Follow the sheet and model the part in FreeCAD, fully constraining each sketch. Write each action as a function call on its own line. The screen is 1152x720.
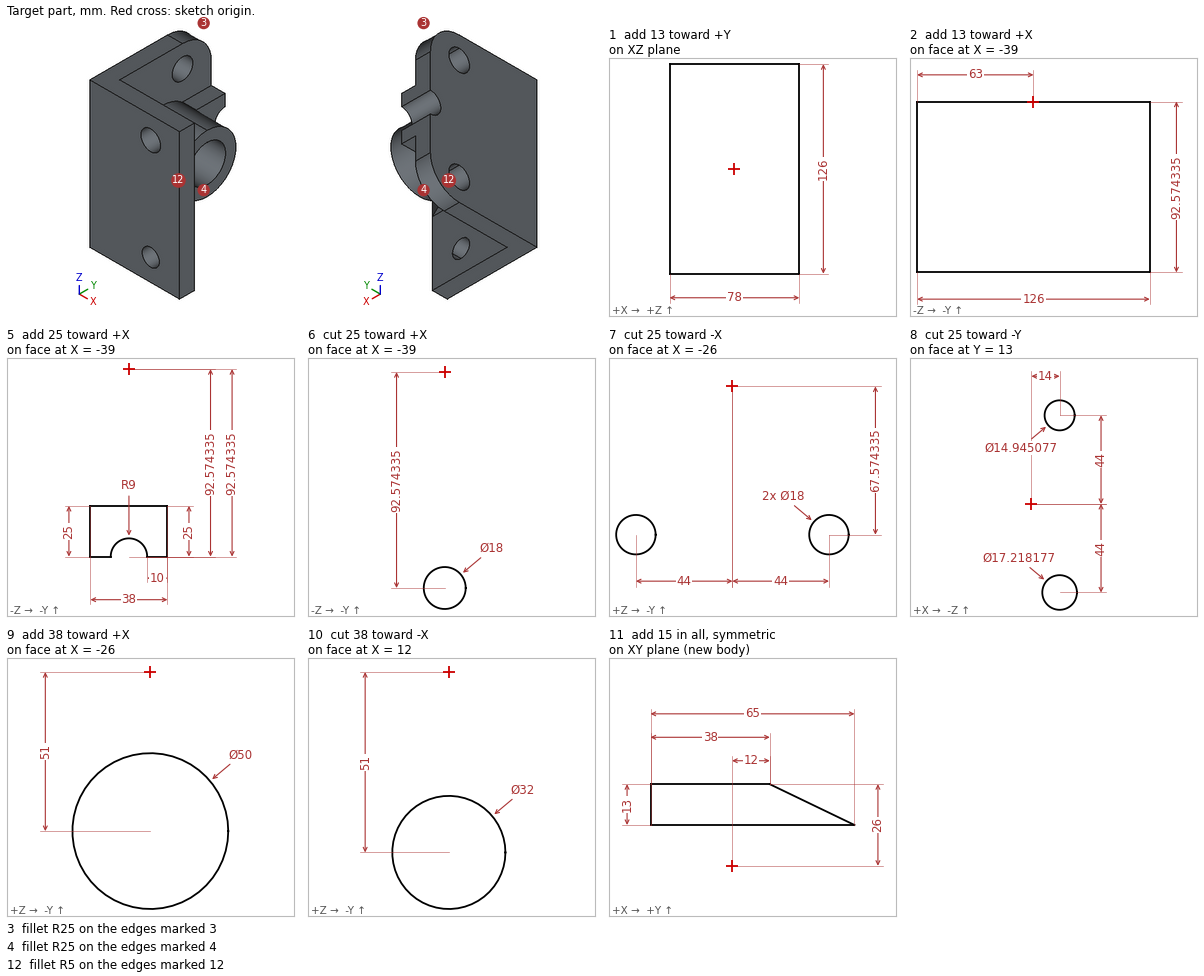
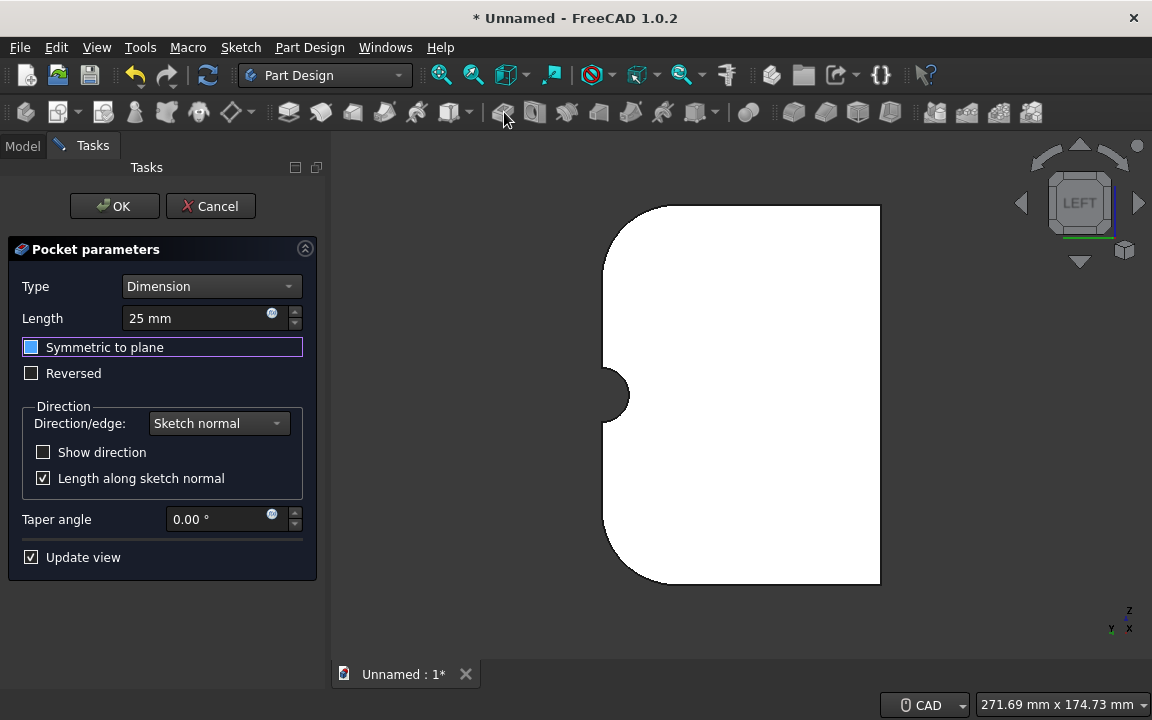
click(115, 206)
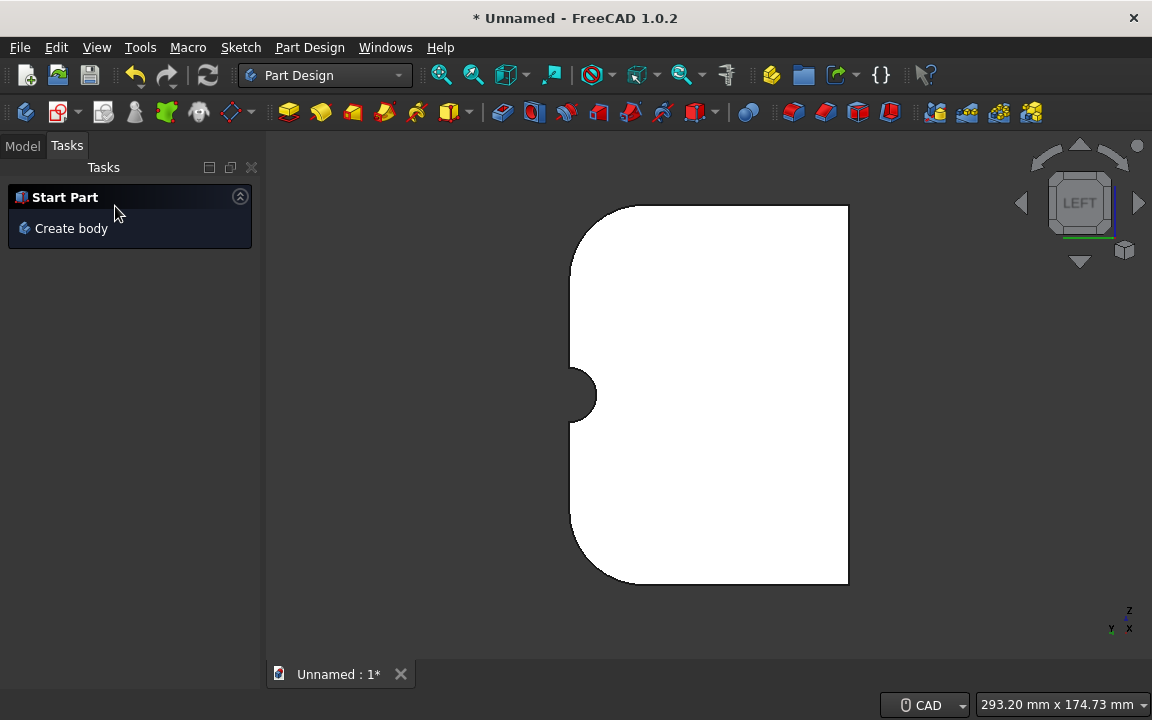
key(0)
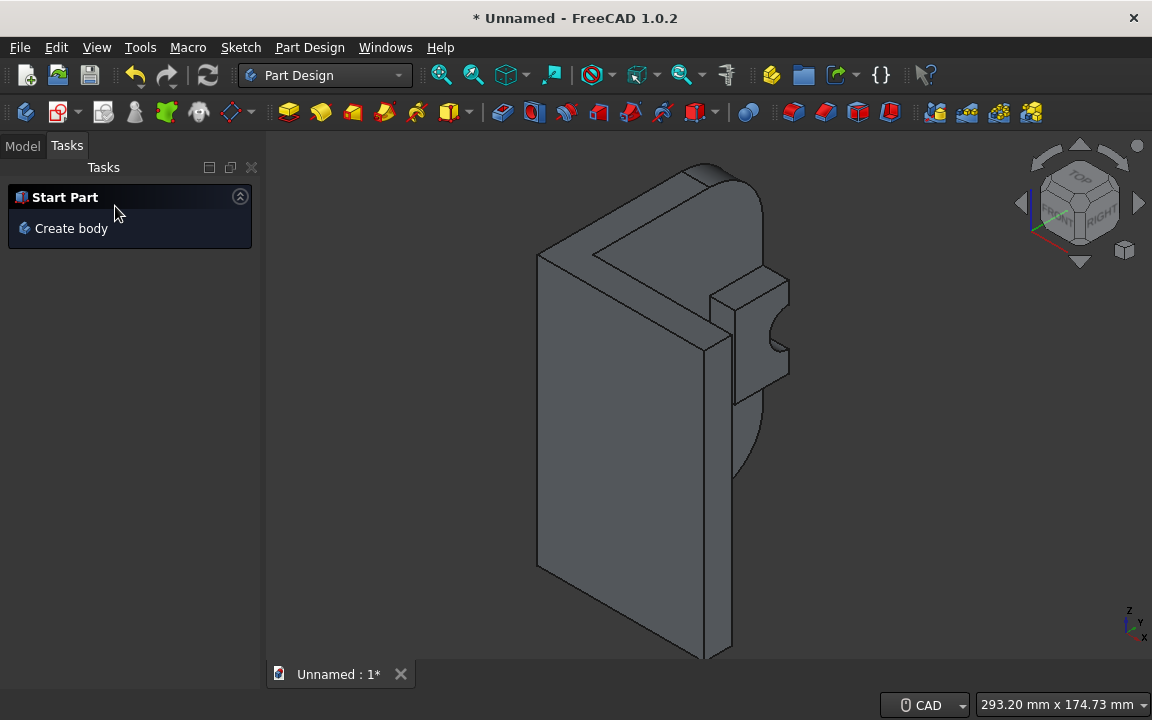
key(v)
key(f)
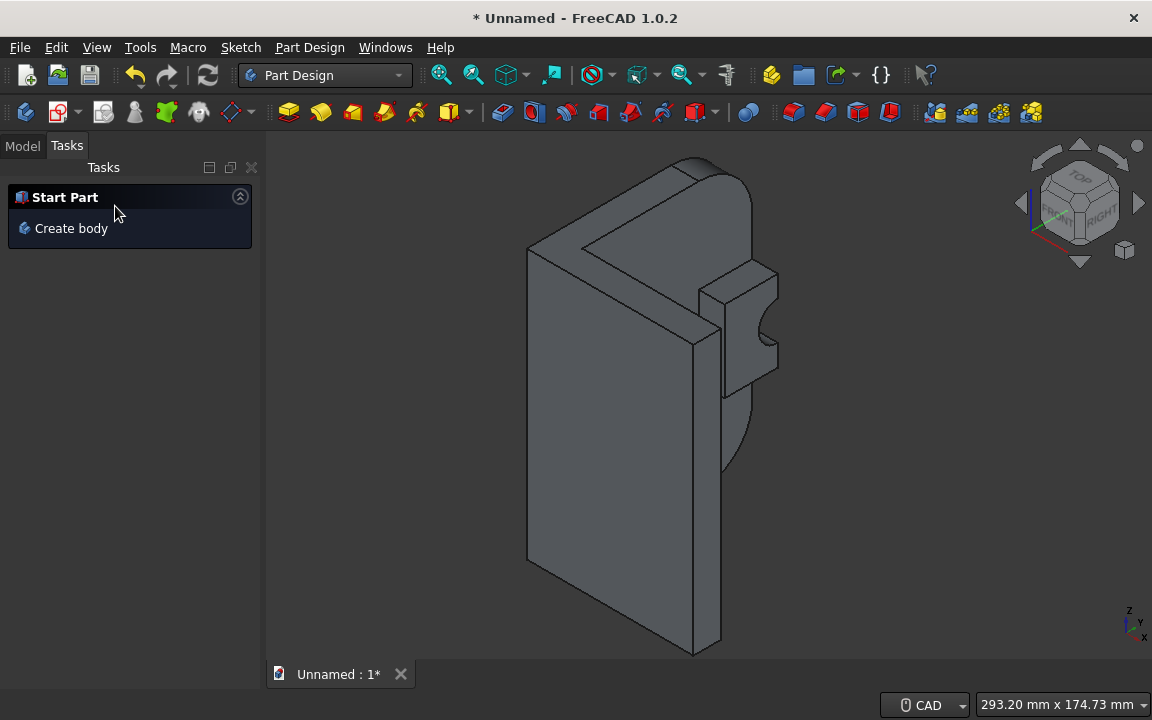
click(667, 265)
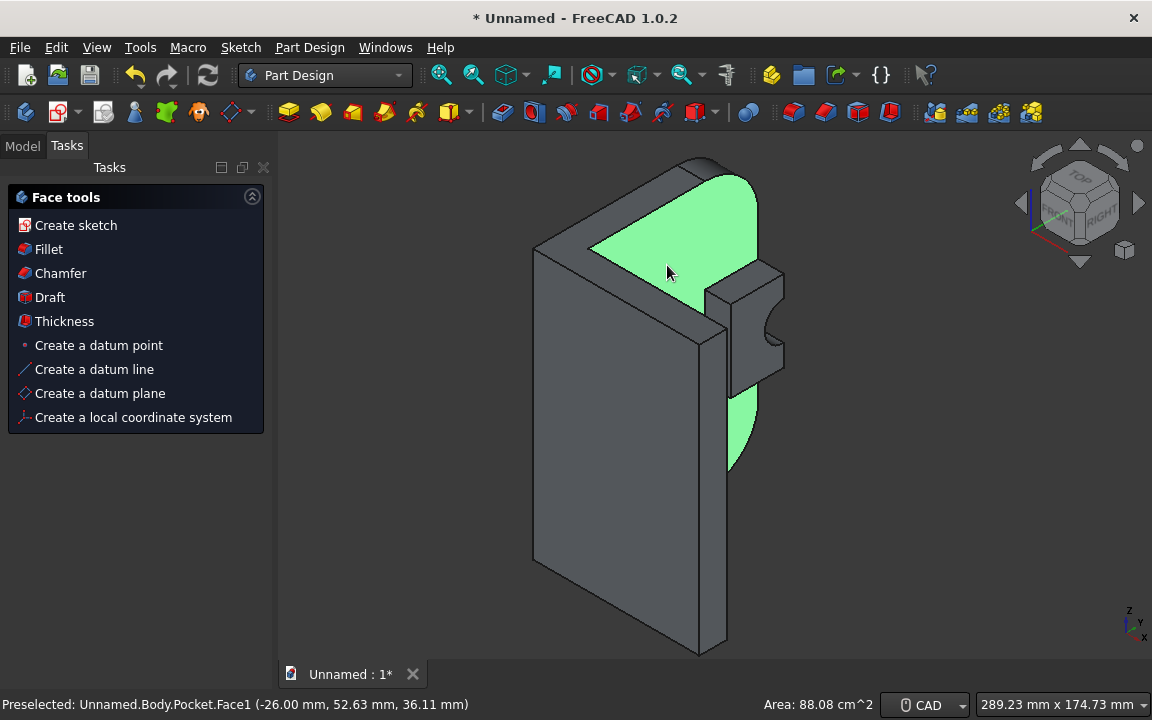
click(58, 112)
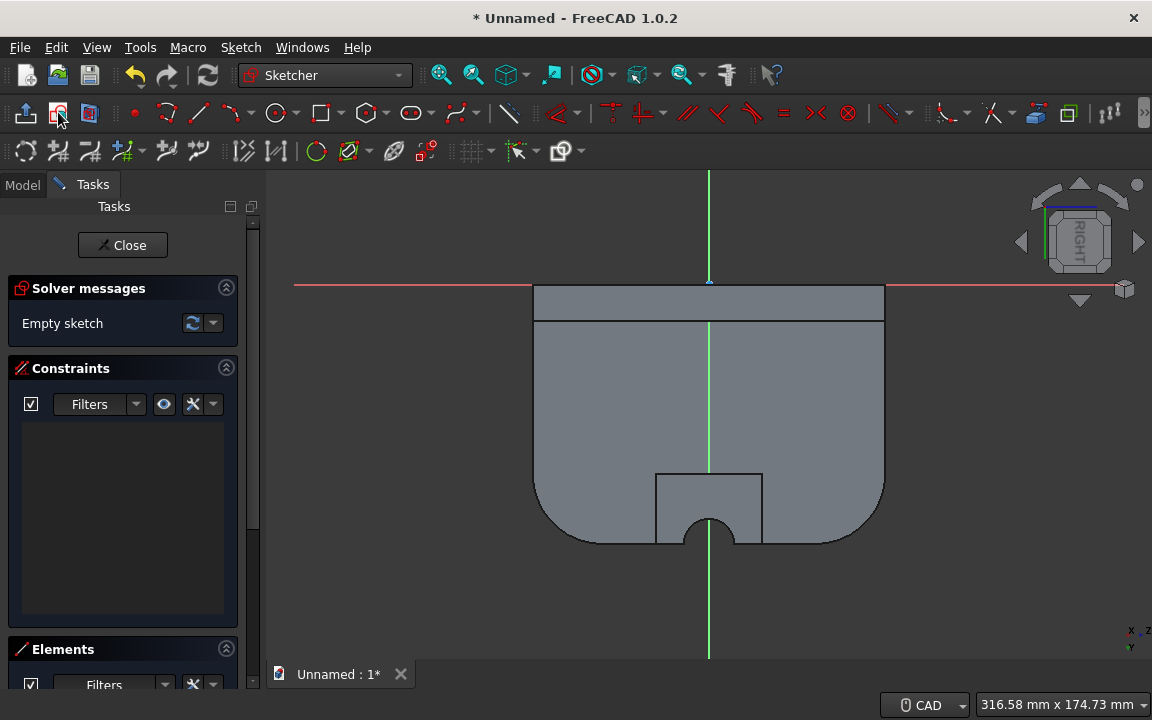
scroll(848, 347, up, 2)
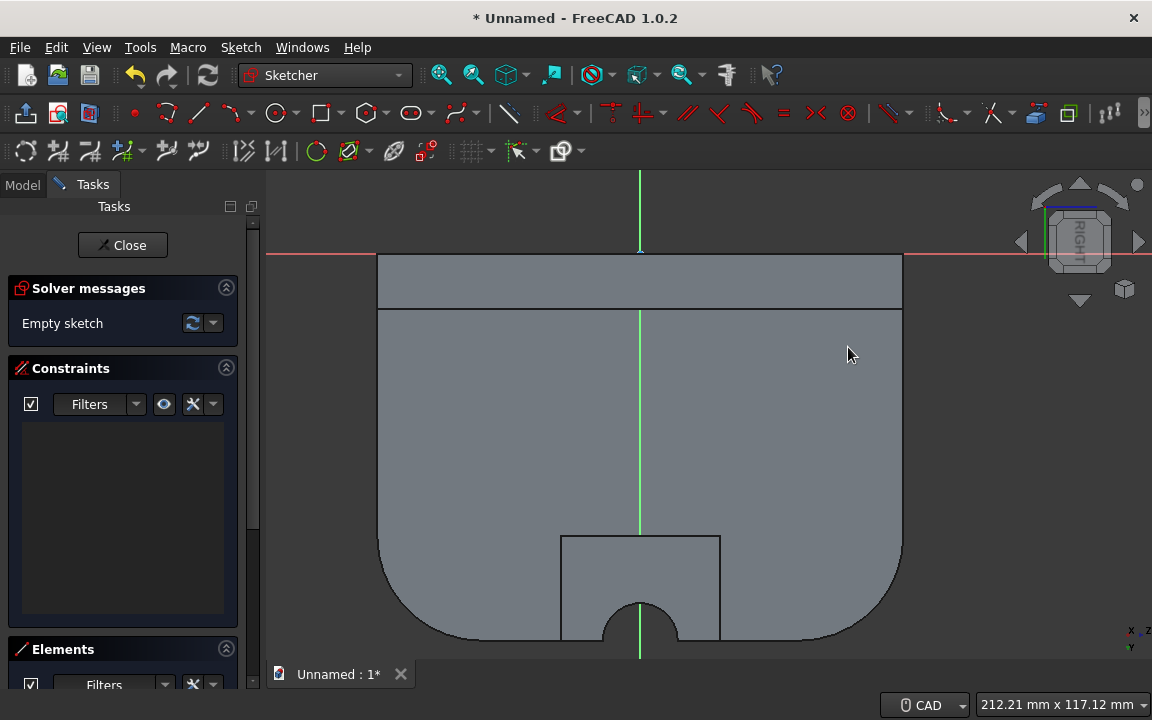
key(g)
key(c)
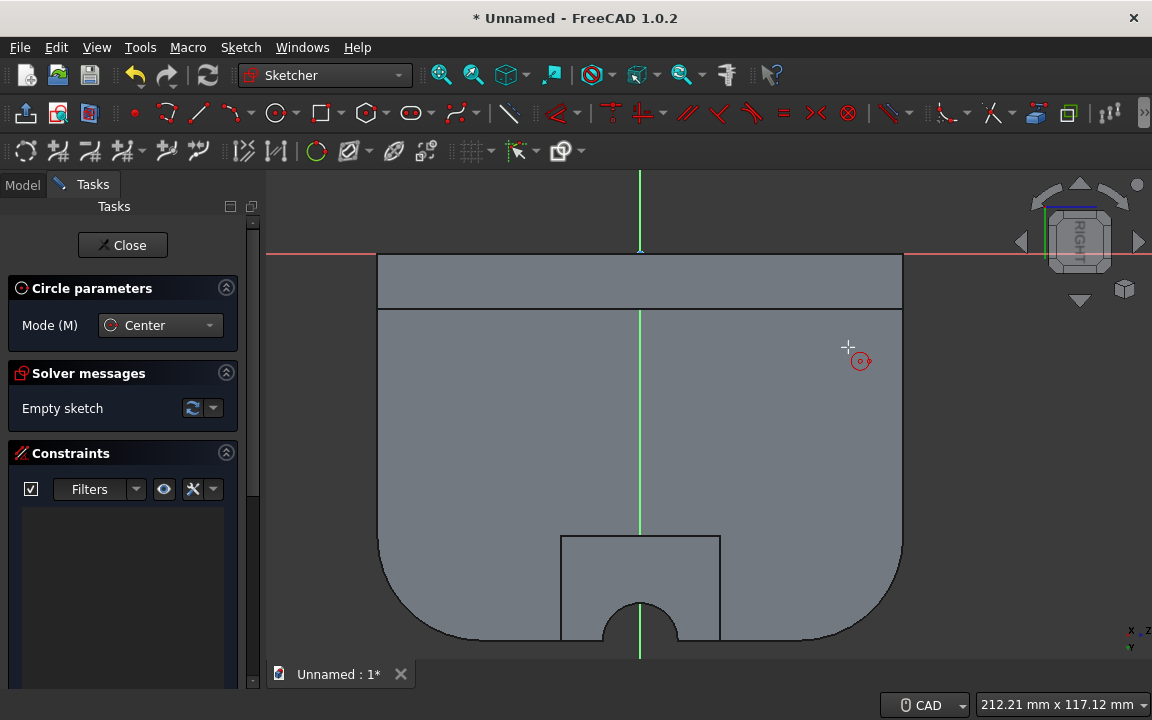
click(824, 536)
move(851, 510)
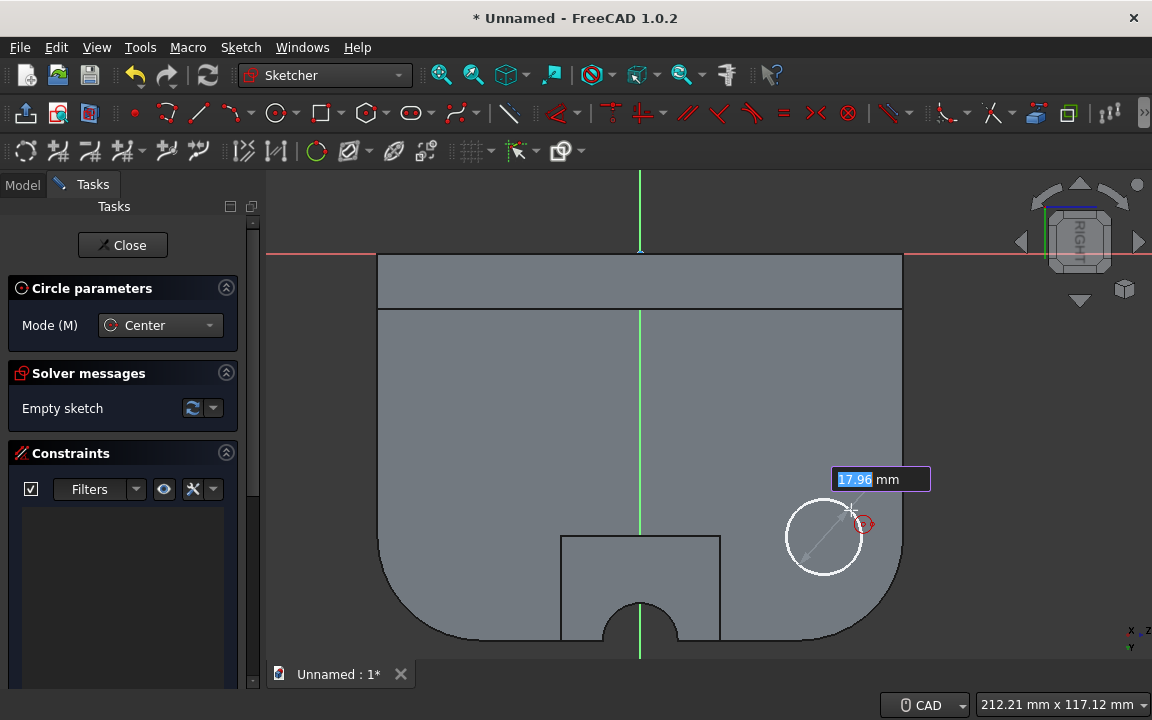
text(18)
key(Return)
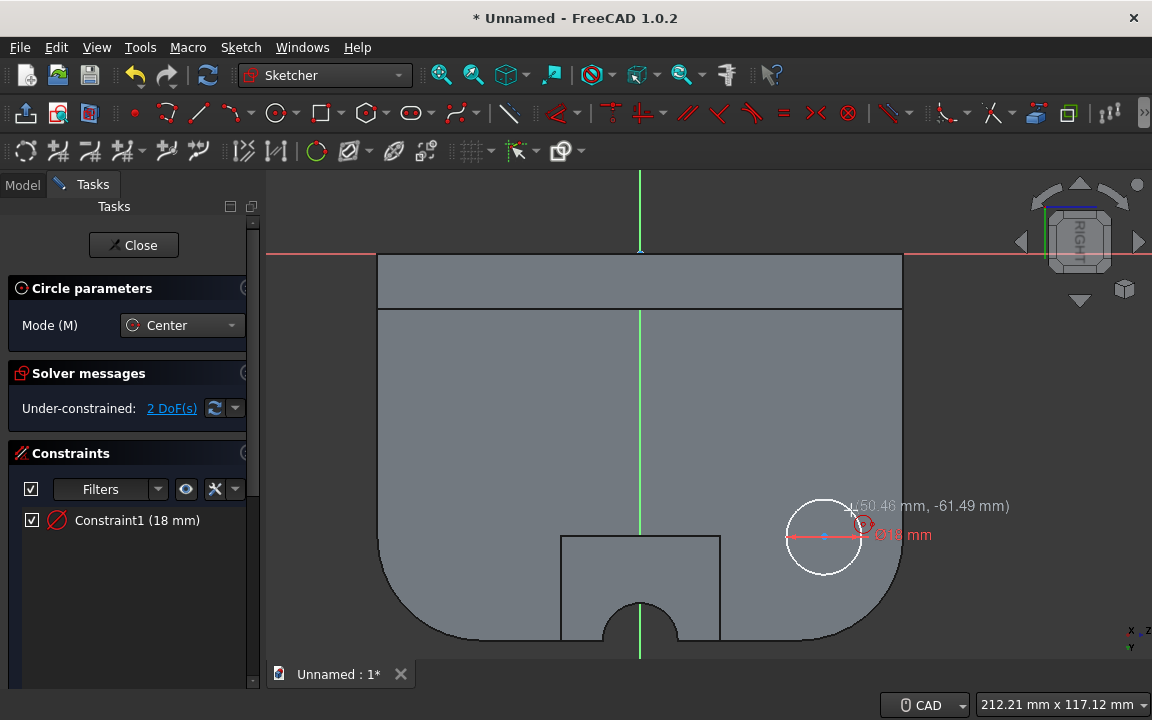
click(457, 536)
move(483, 510)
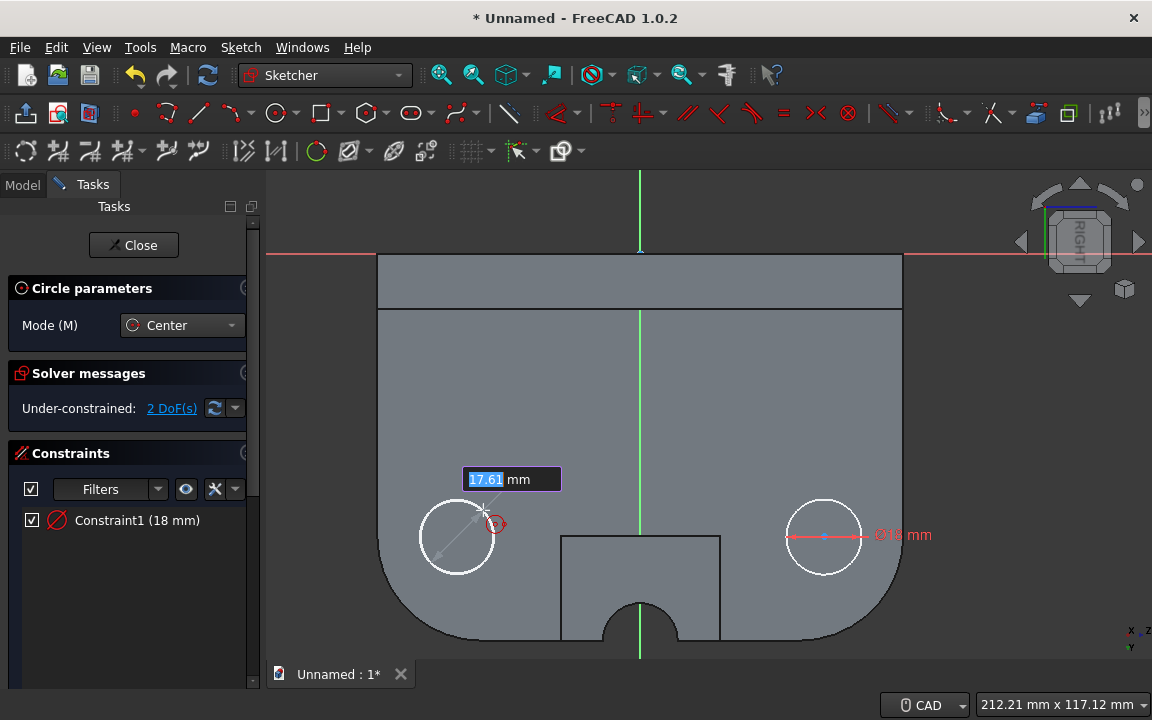
text(18)
key(Return)
key(Escape)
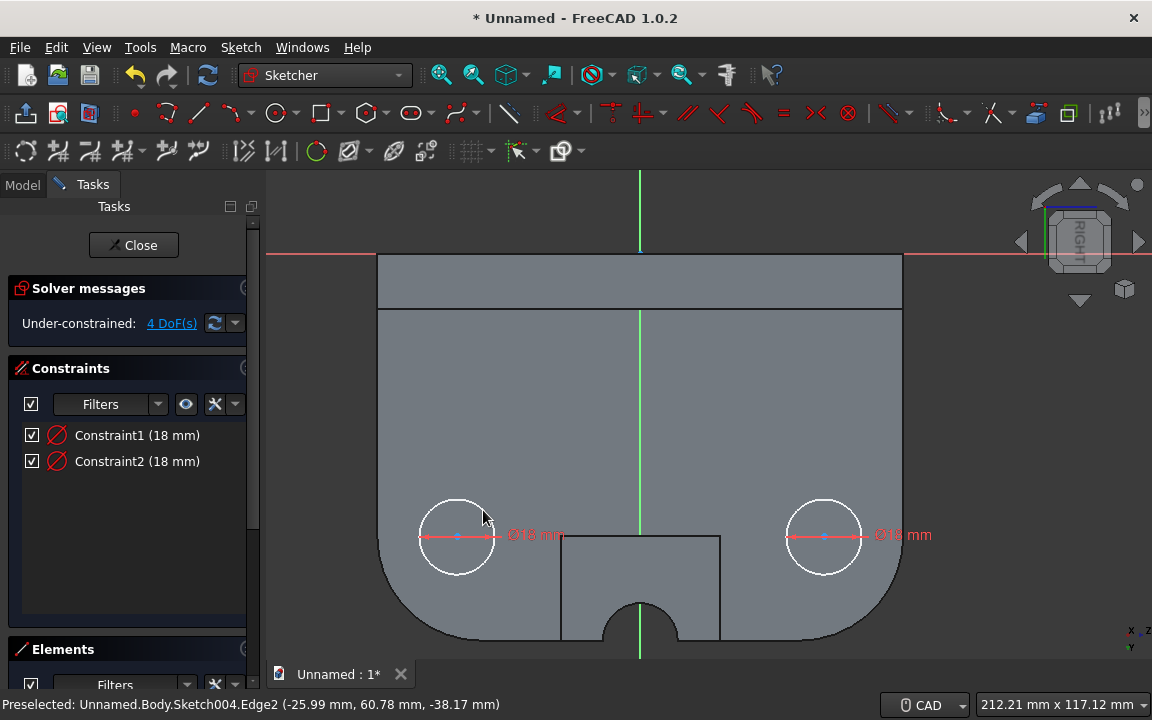
click(824, 537)